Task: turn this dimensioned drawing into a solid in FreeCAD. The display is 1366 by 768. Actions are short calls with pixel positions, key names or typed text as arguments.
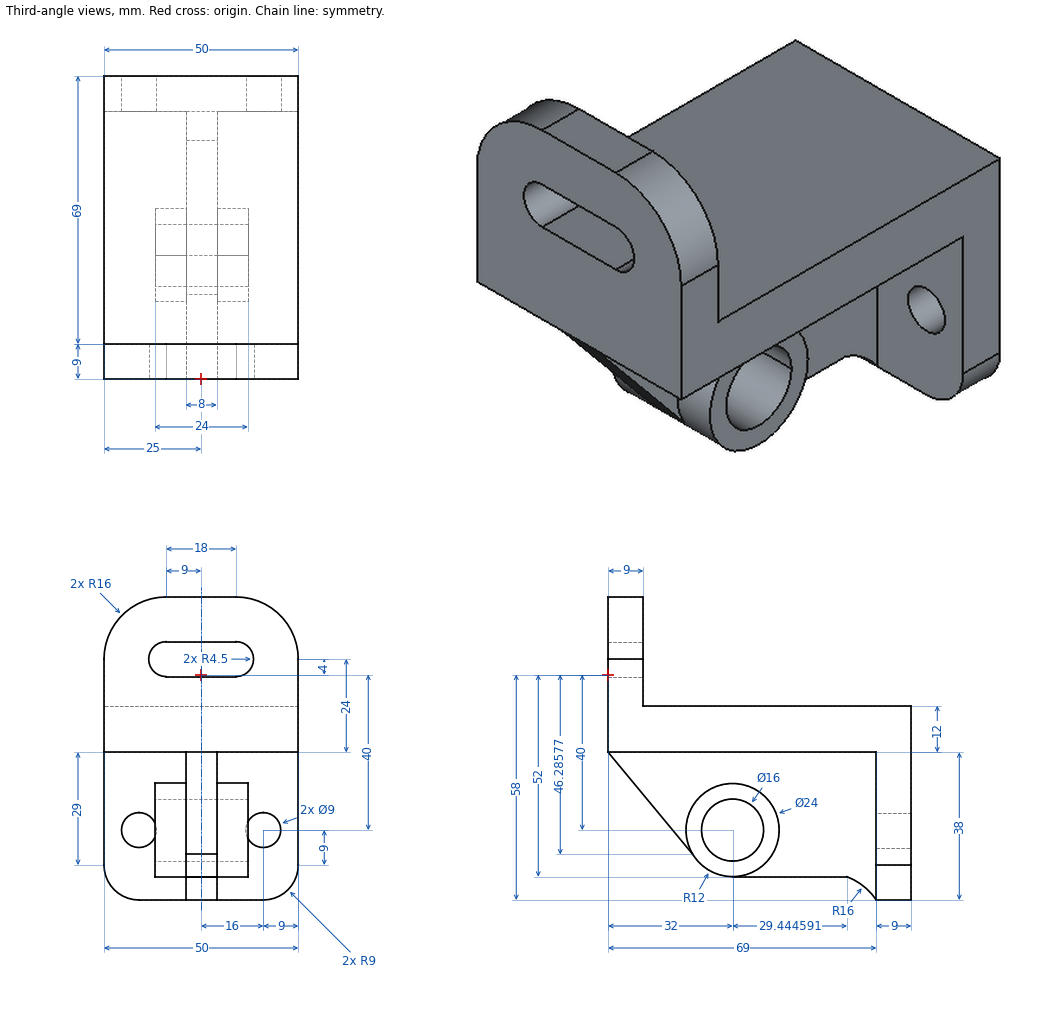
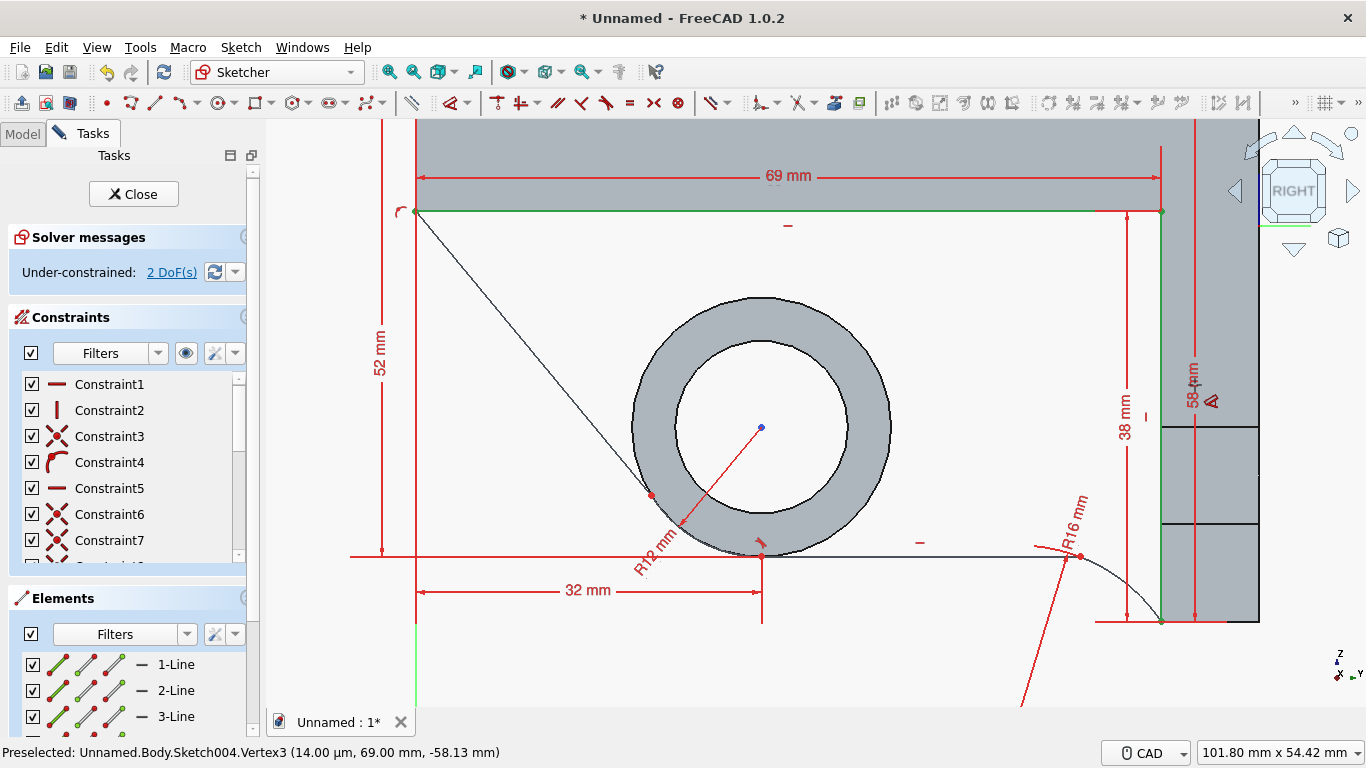
click(857, 557)
click(921, 591)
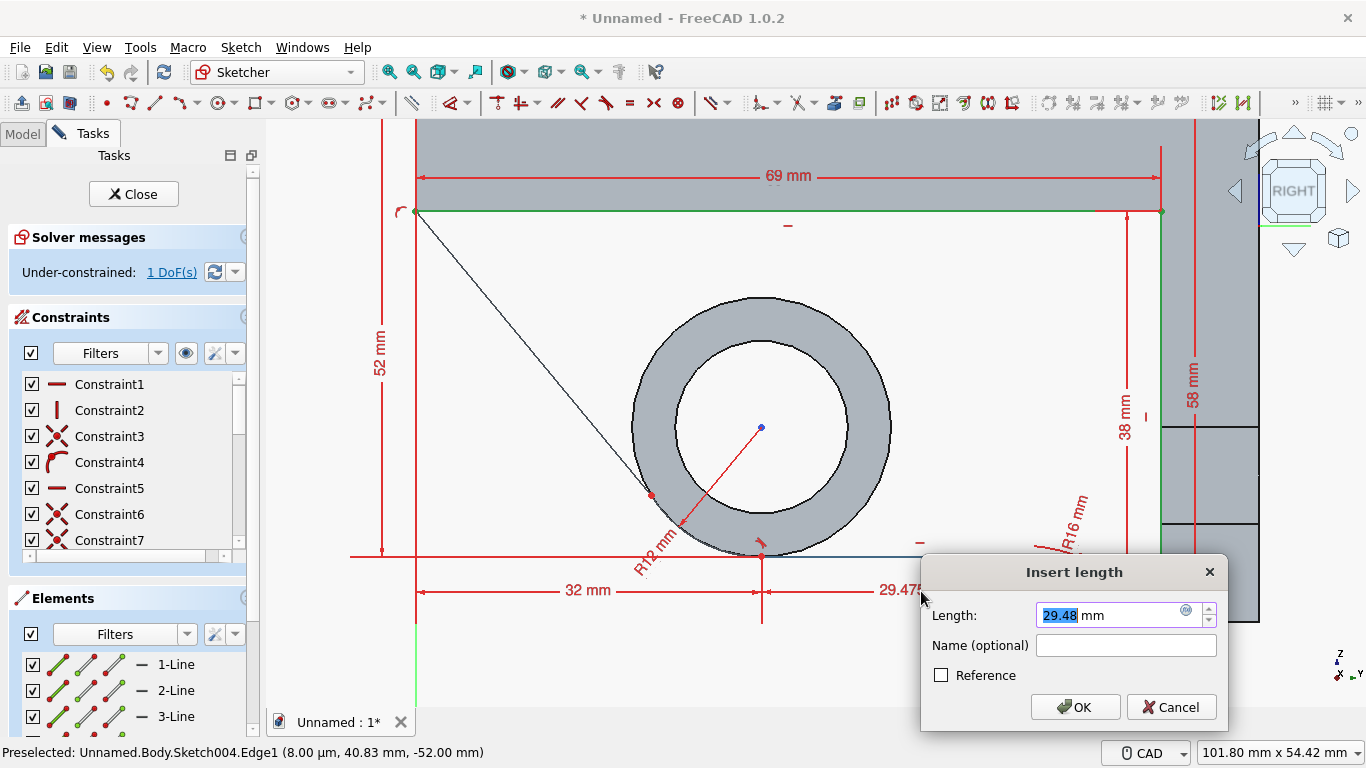
text(29.444591)
key(Return)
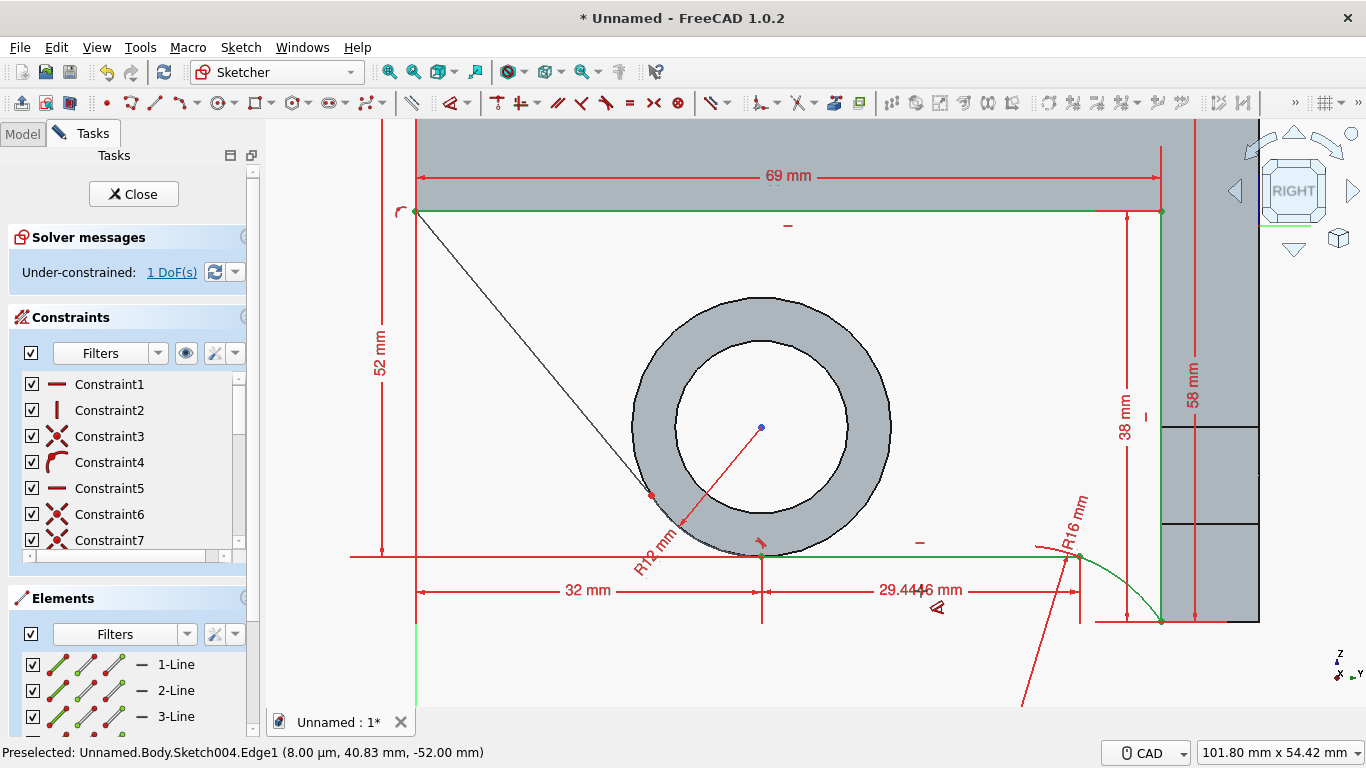
click(652, 496)
click(382, 321)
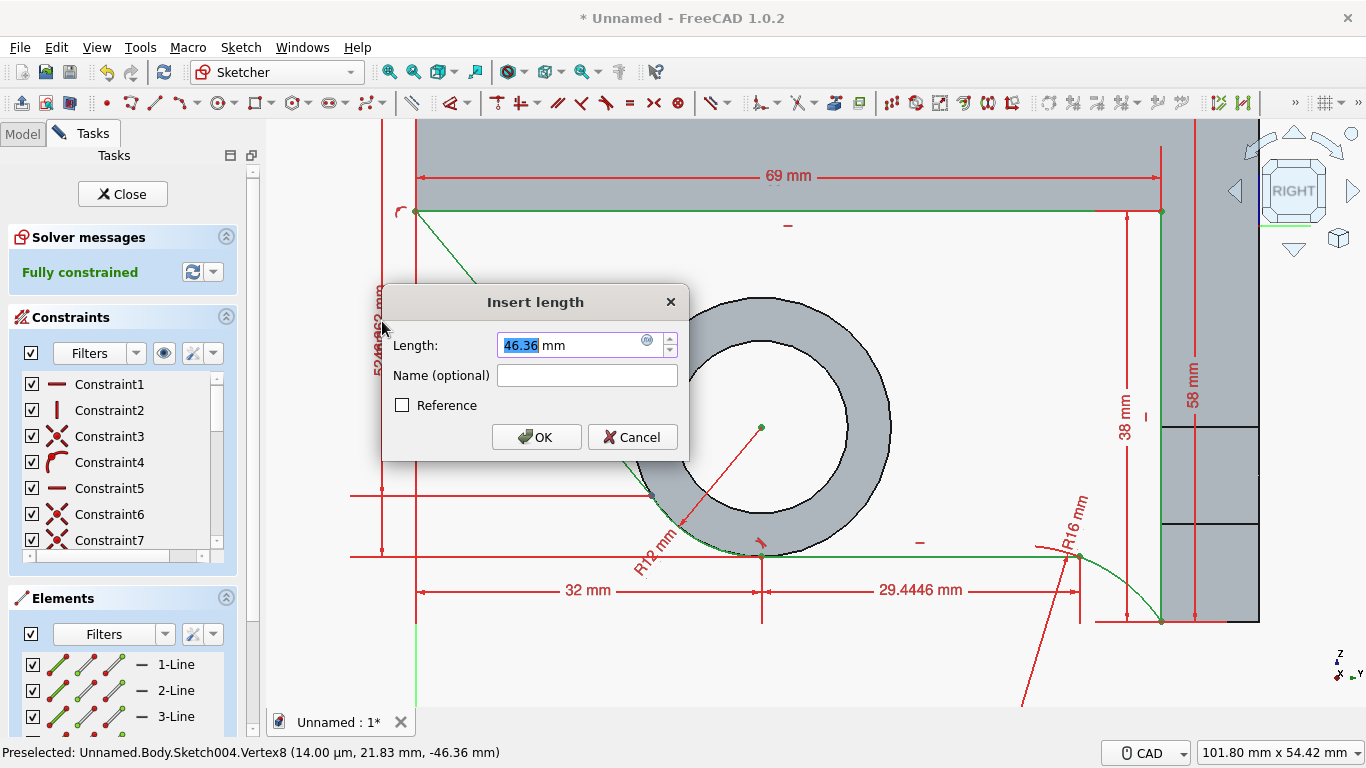
text(46.28577)
key(Return)
key(Escape)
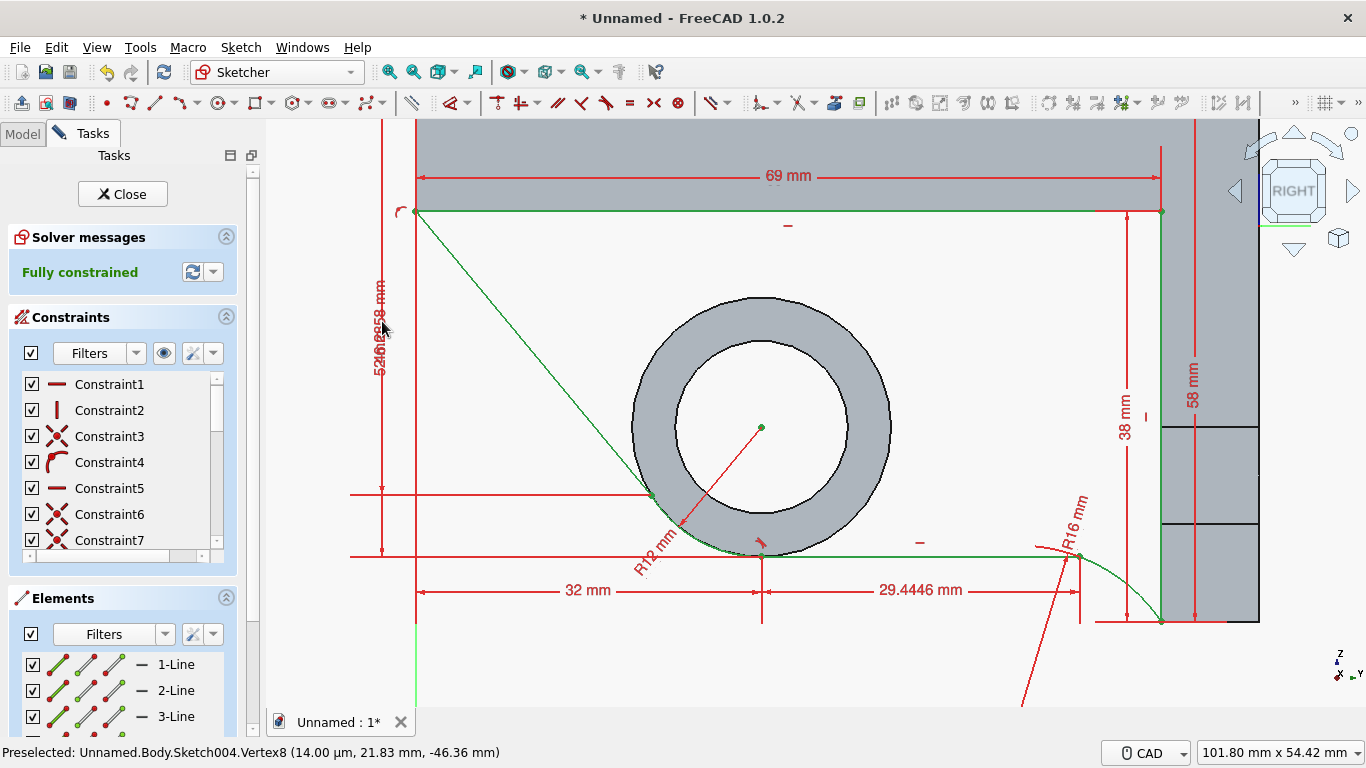
click(123, 194)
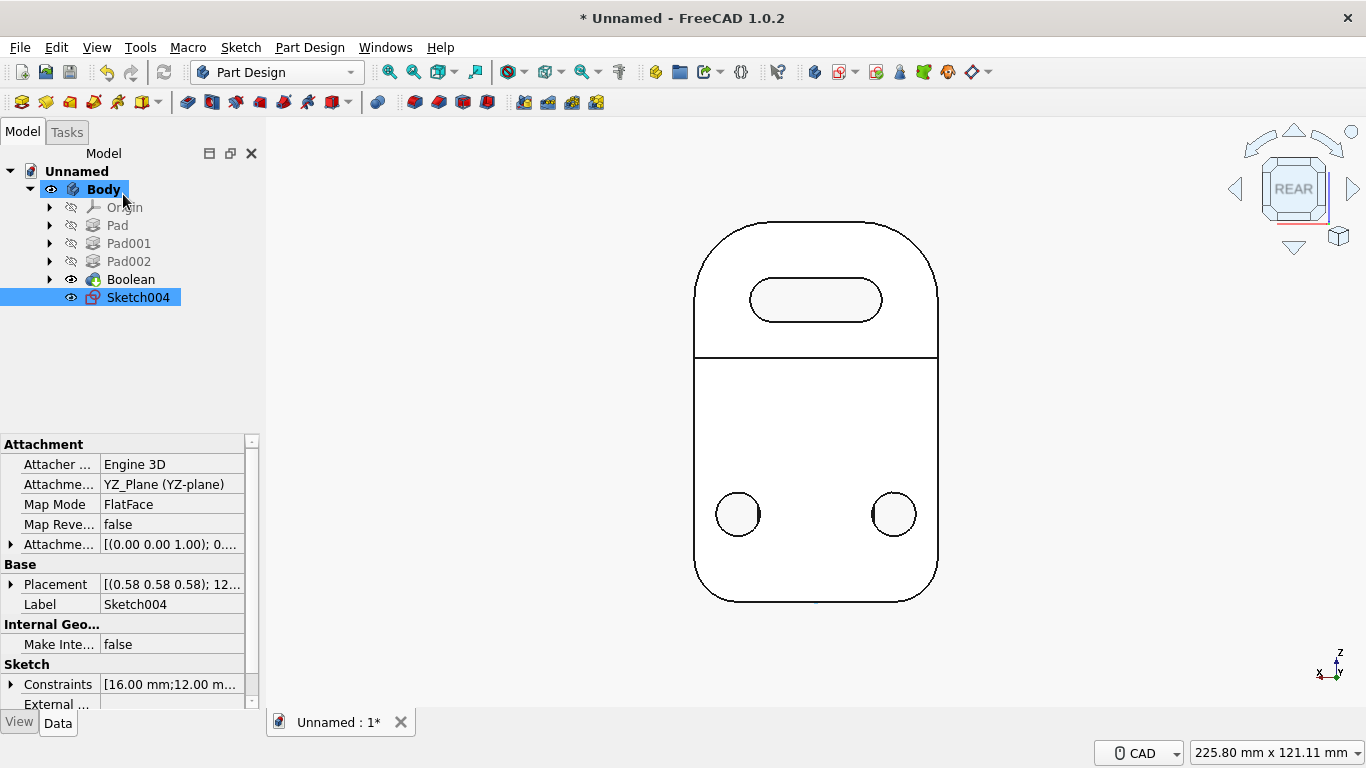
click(22, 102)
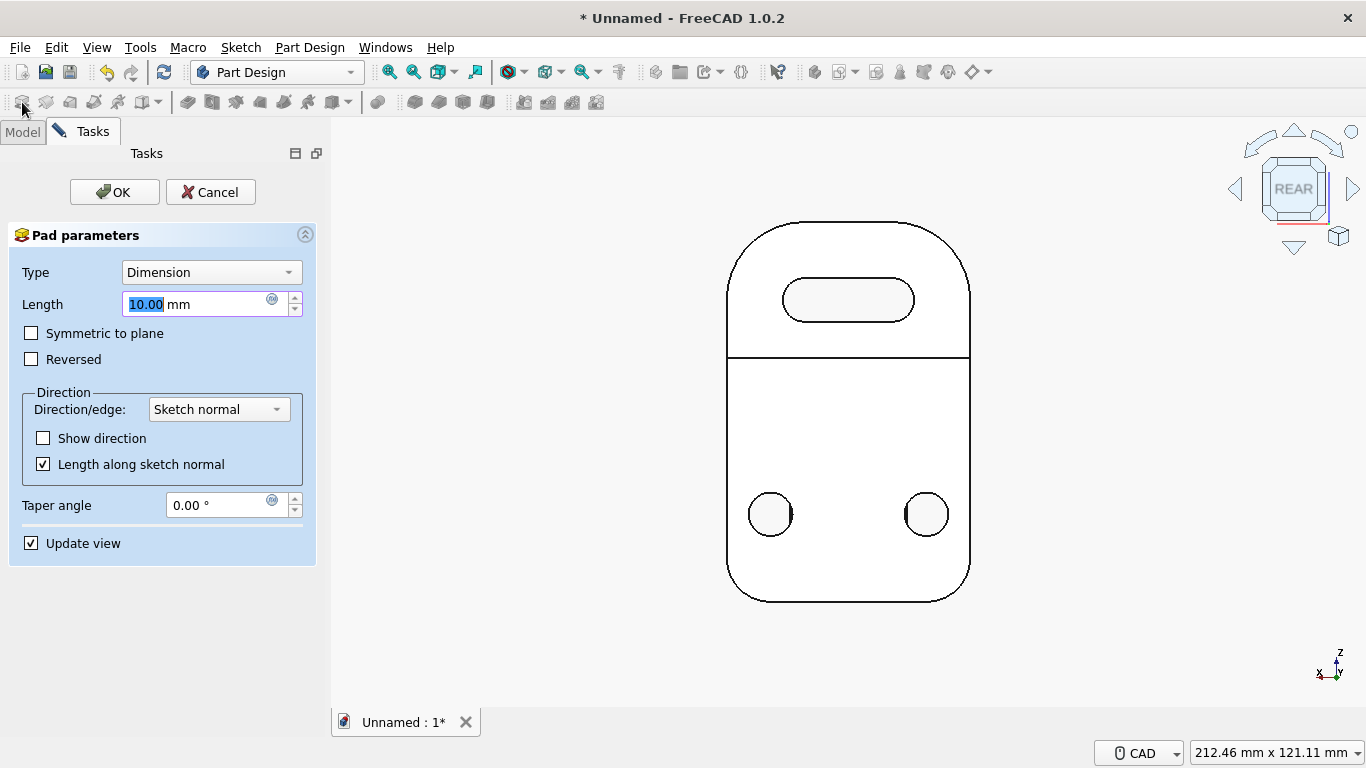
text(8)
key(Tab)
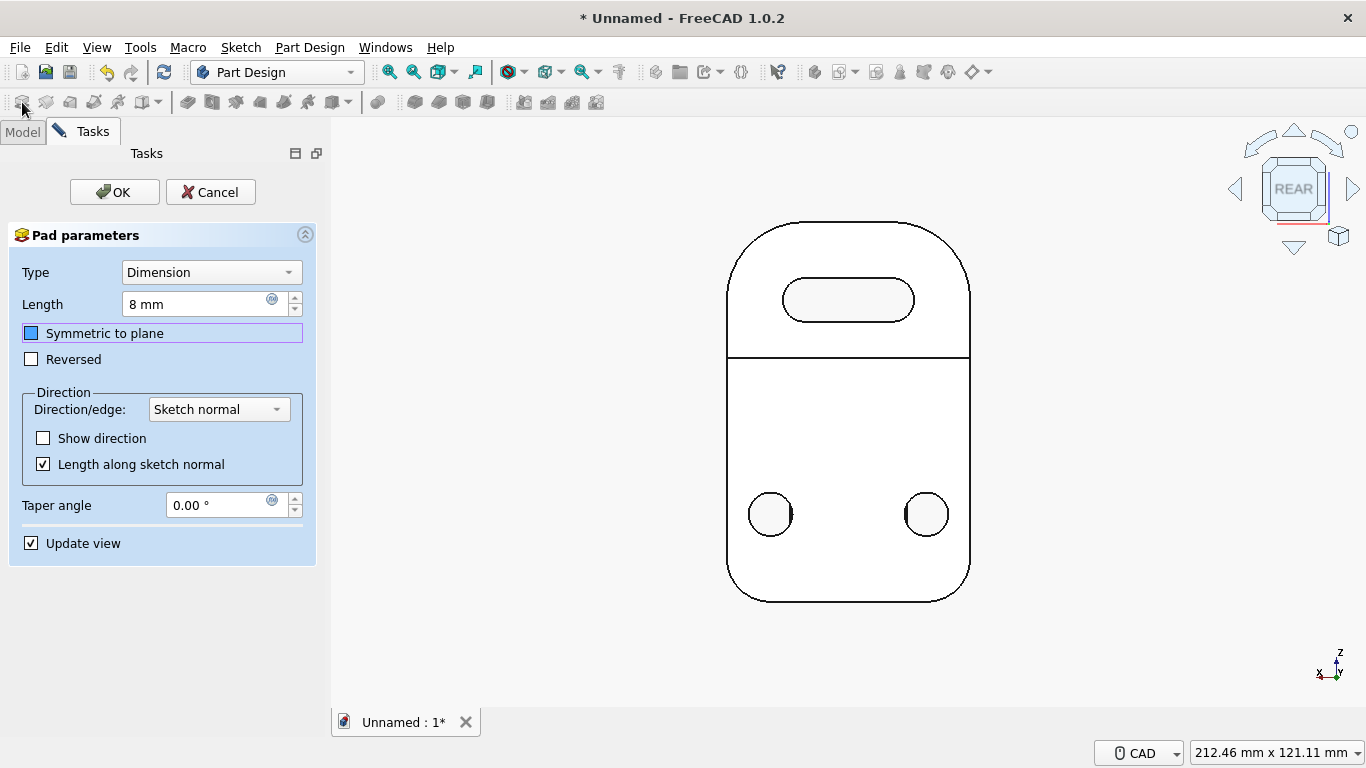
click(30, 333)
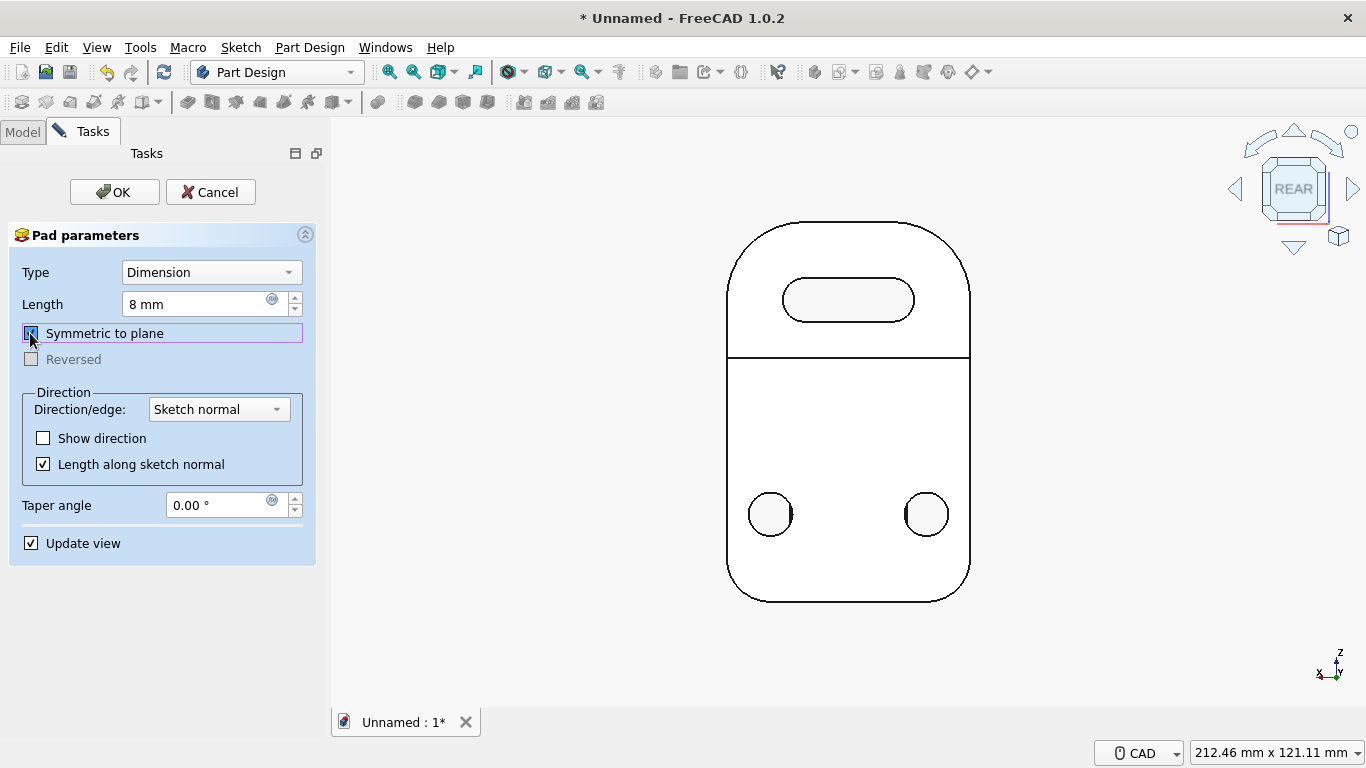
click(115, 192)